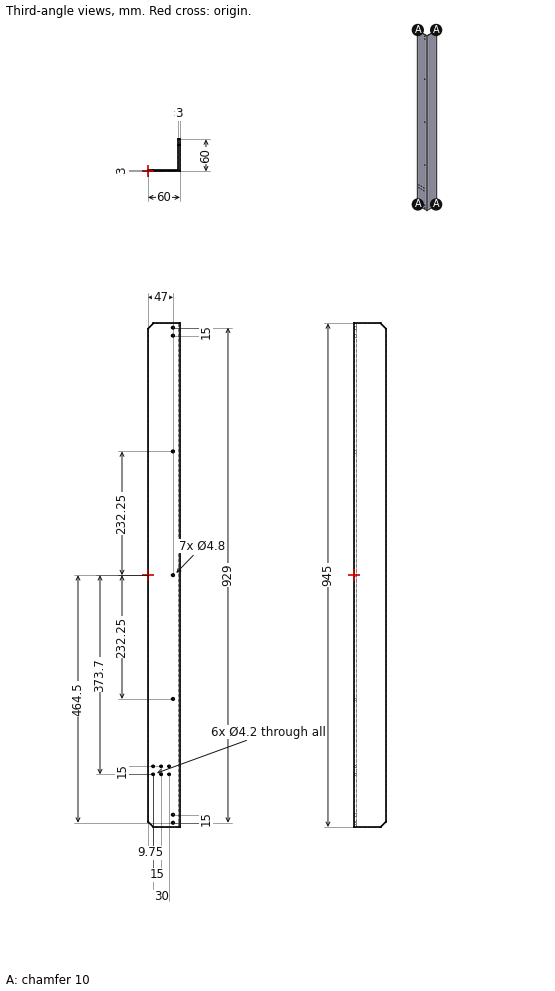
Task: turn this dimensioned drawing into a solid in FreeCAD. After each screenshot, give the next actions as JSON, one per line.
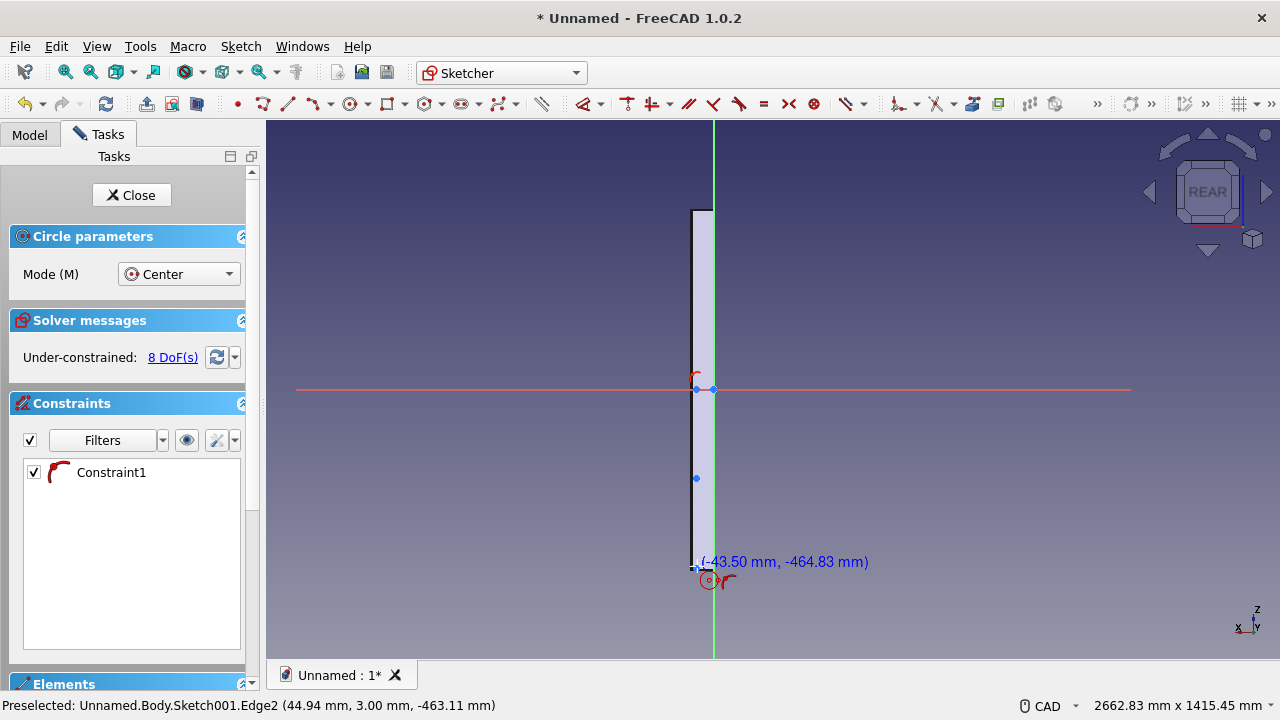
{"action": "scroll", "coordinate": [696, 213], "scroll_direction": "up", "scroll_amount": 17}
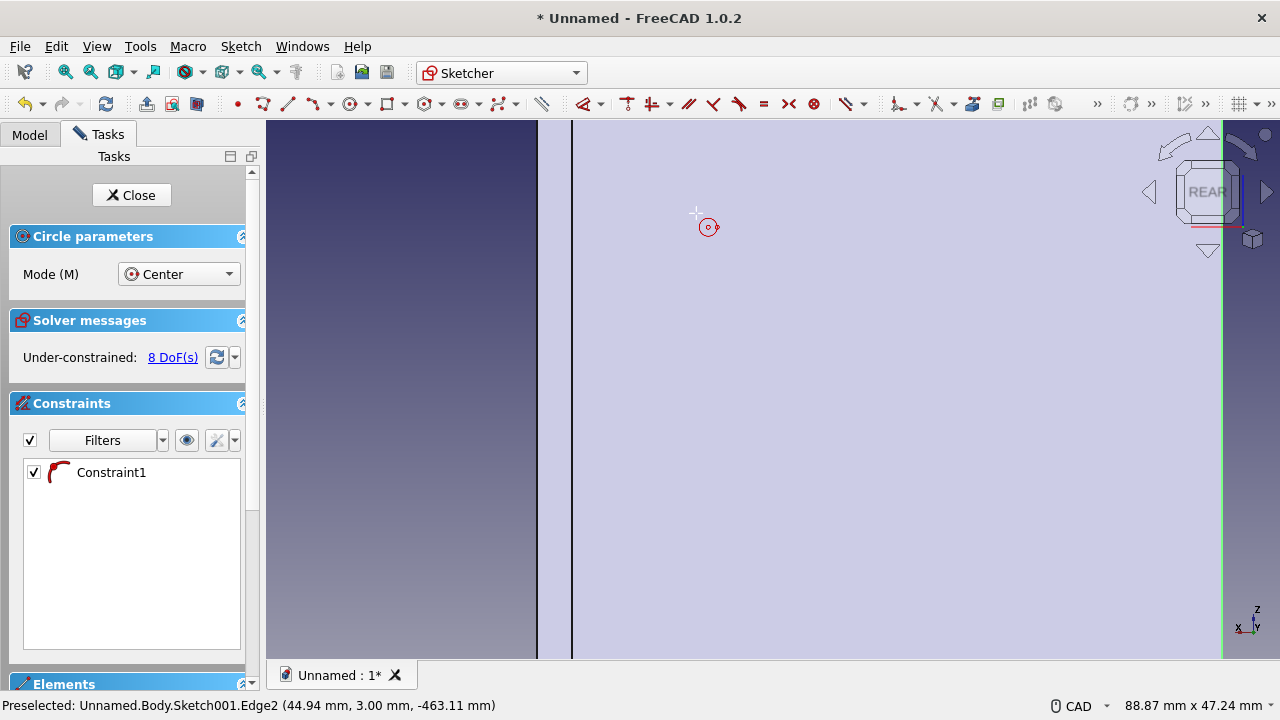
{"action": "scroll", "coordinate": [696, 213], "scroll_direction": "down", "scroll_amount": 17}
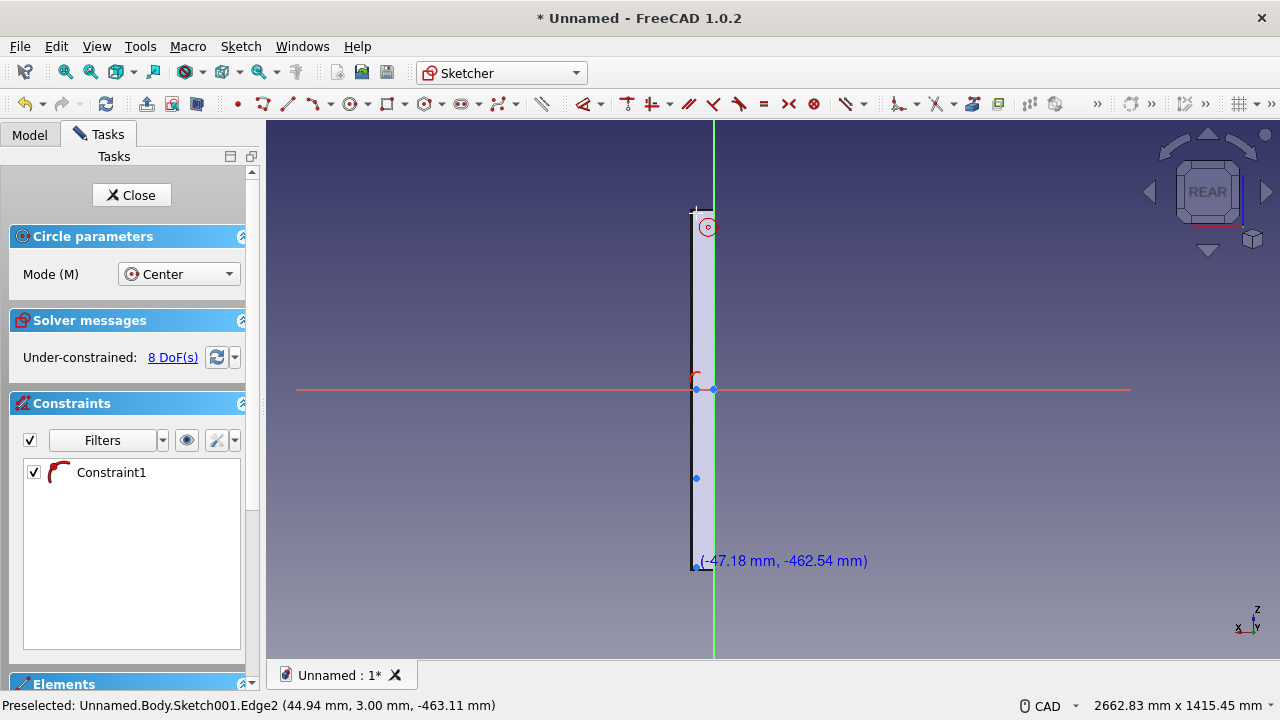
{"action": "left_click", "coordinate": [696, 213]}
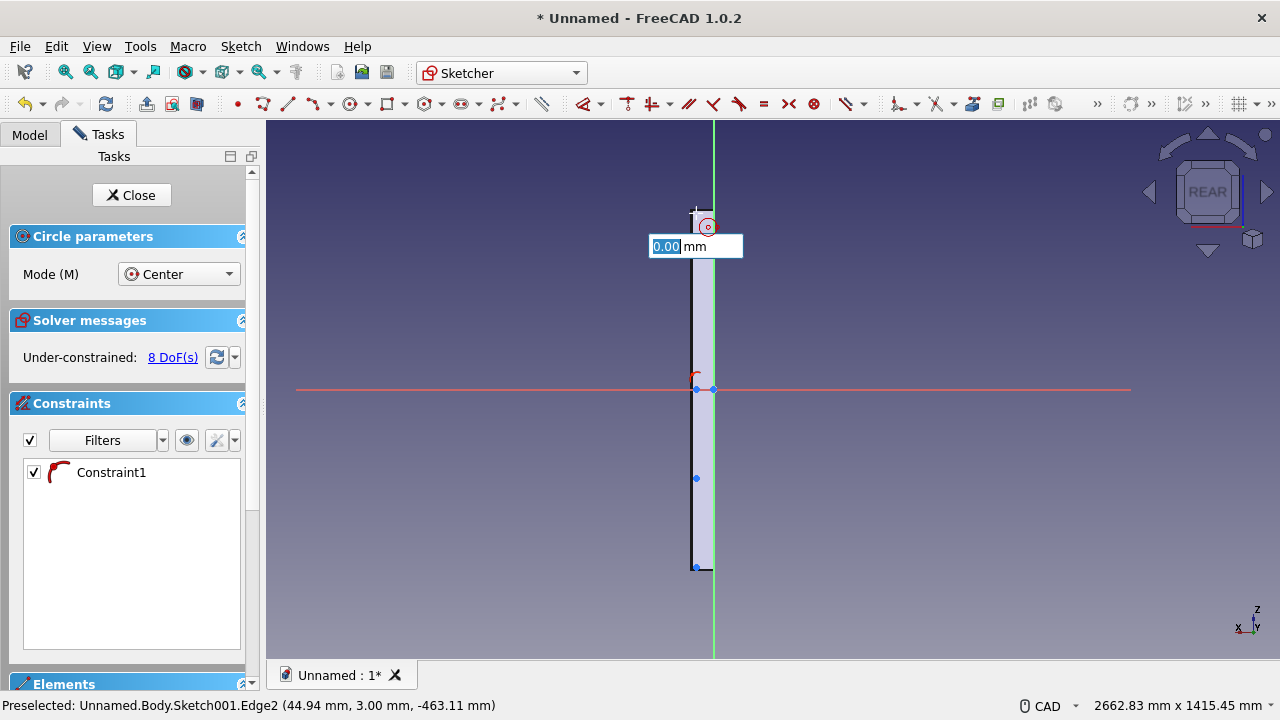
{"action": "scroll", "coordinate": [697, 212], "scroll_direction": "up", "scroll_amount": 15}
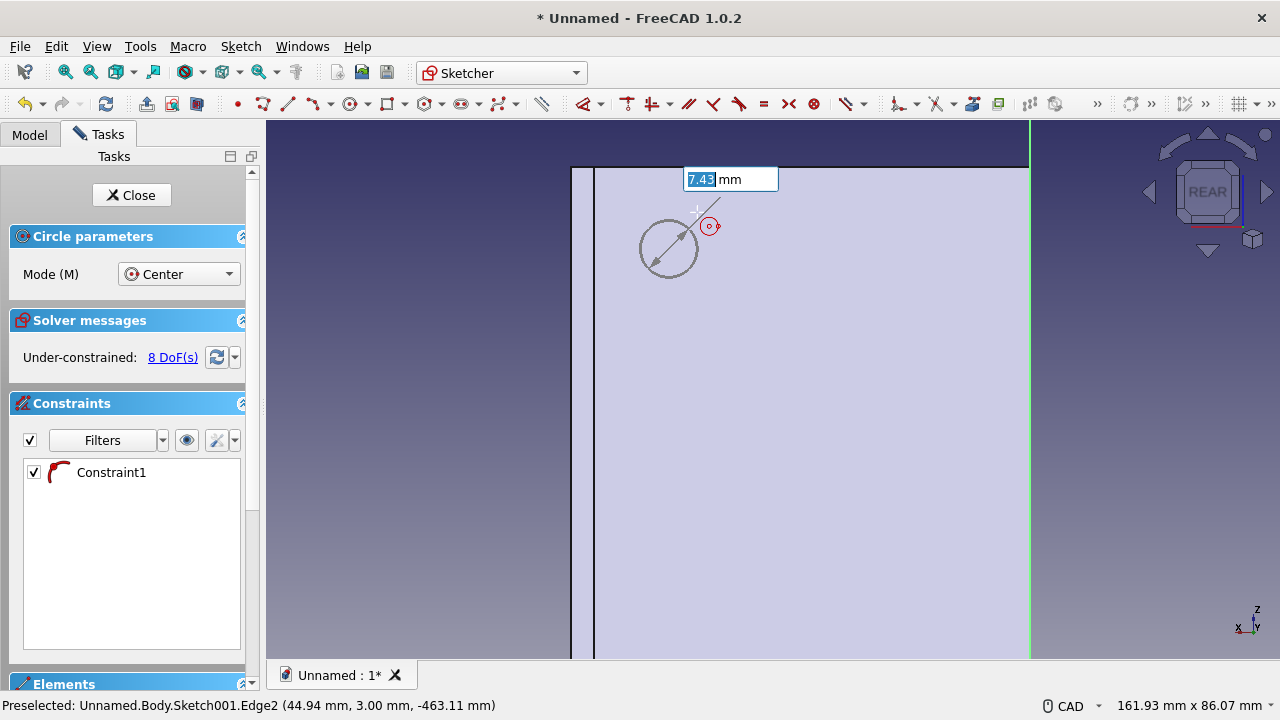
{"action": "left_click", "coordinate": [683, 215]}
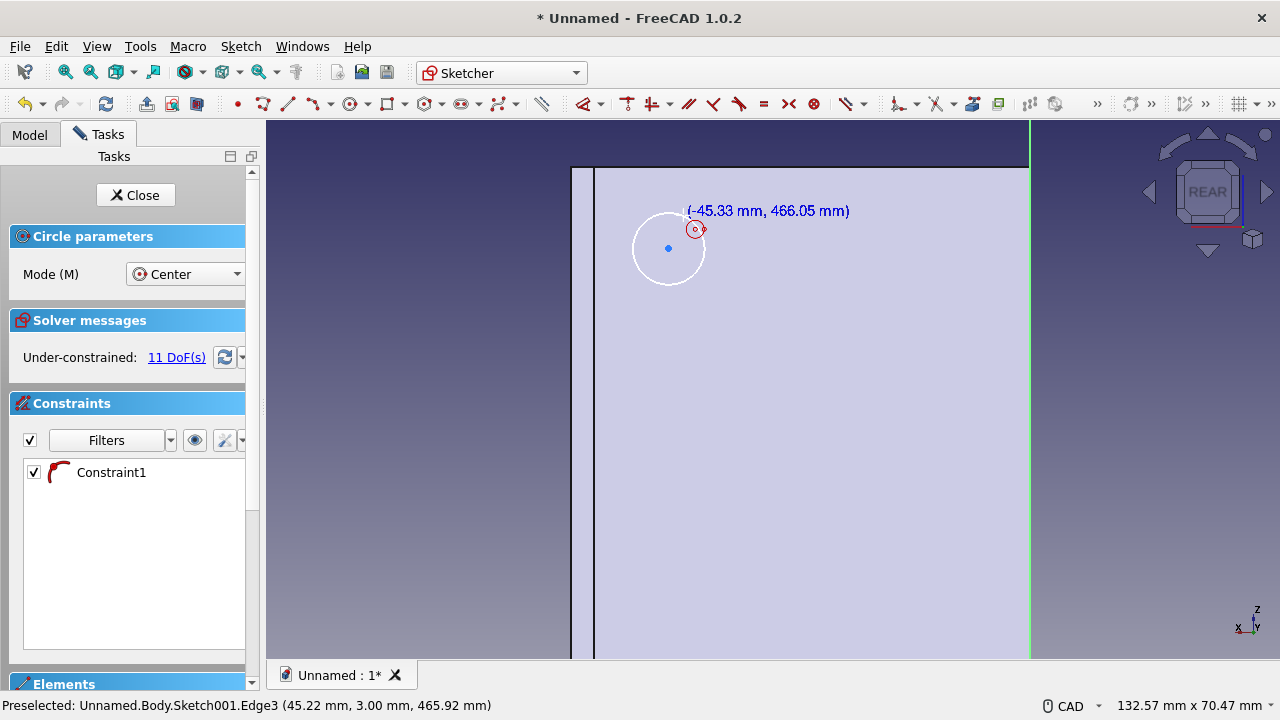
{"action": "scroll", "coordinate": [697, 212], "scroll_direction": "down", "scroll_amount": 15}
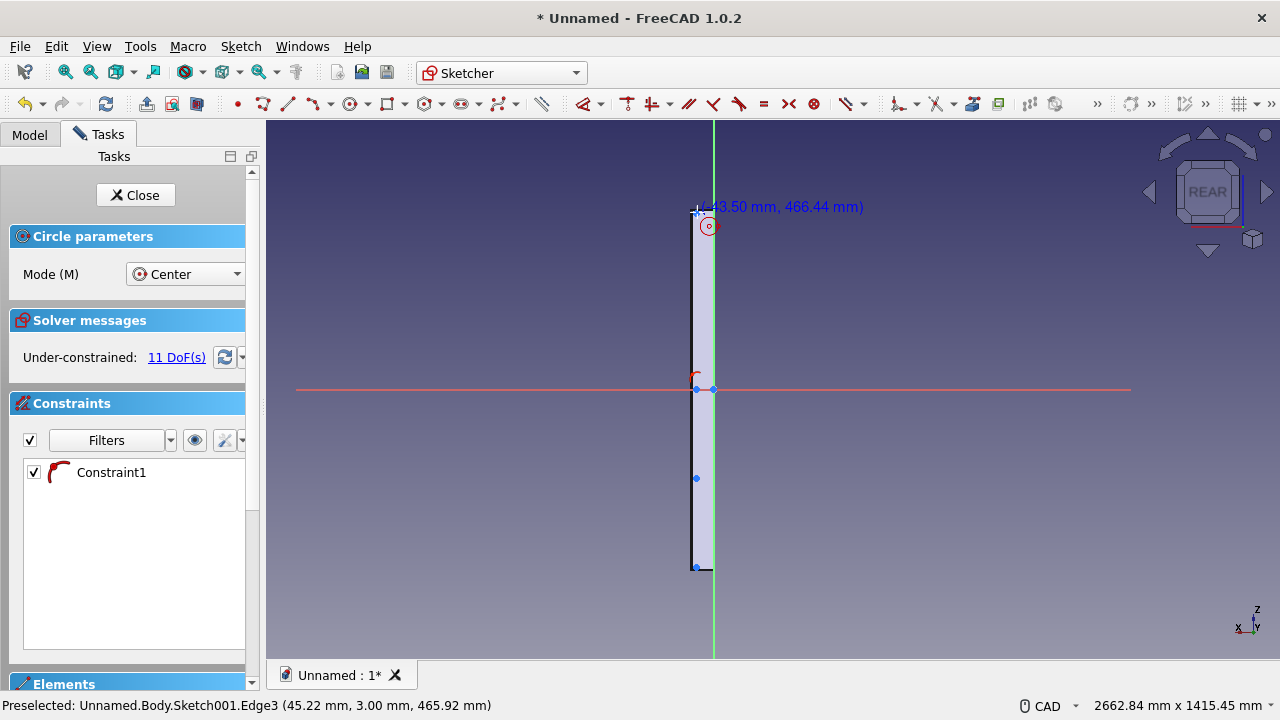
{"action": "scroll", "coordinate": [696, 301], "scroll_direction": "up", "scroll_amount": 17}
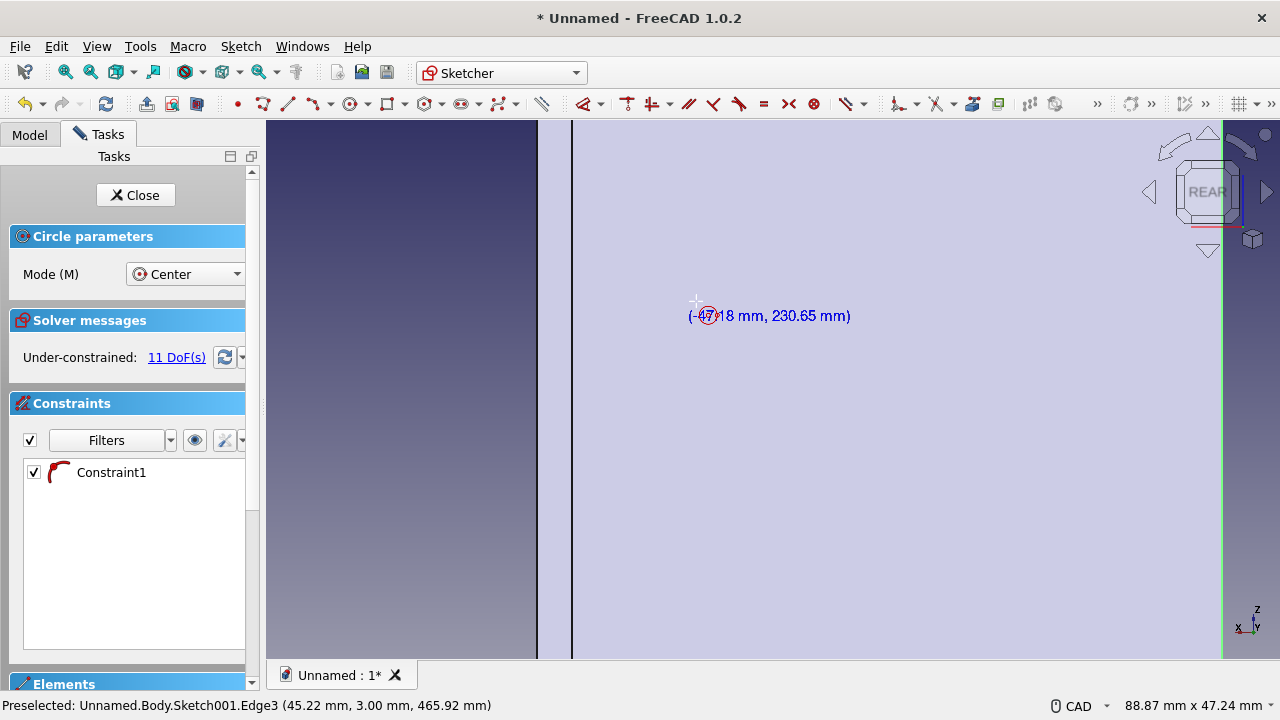
{"action": "scroll", "coordinate": [696, 301], "scroll_direction": "down", "scroll_amount": 17}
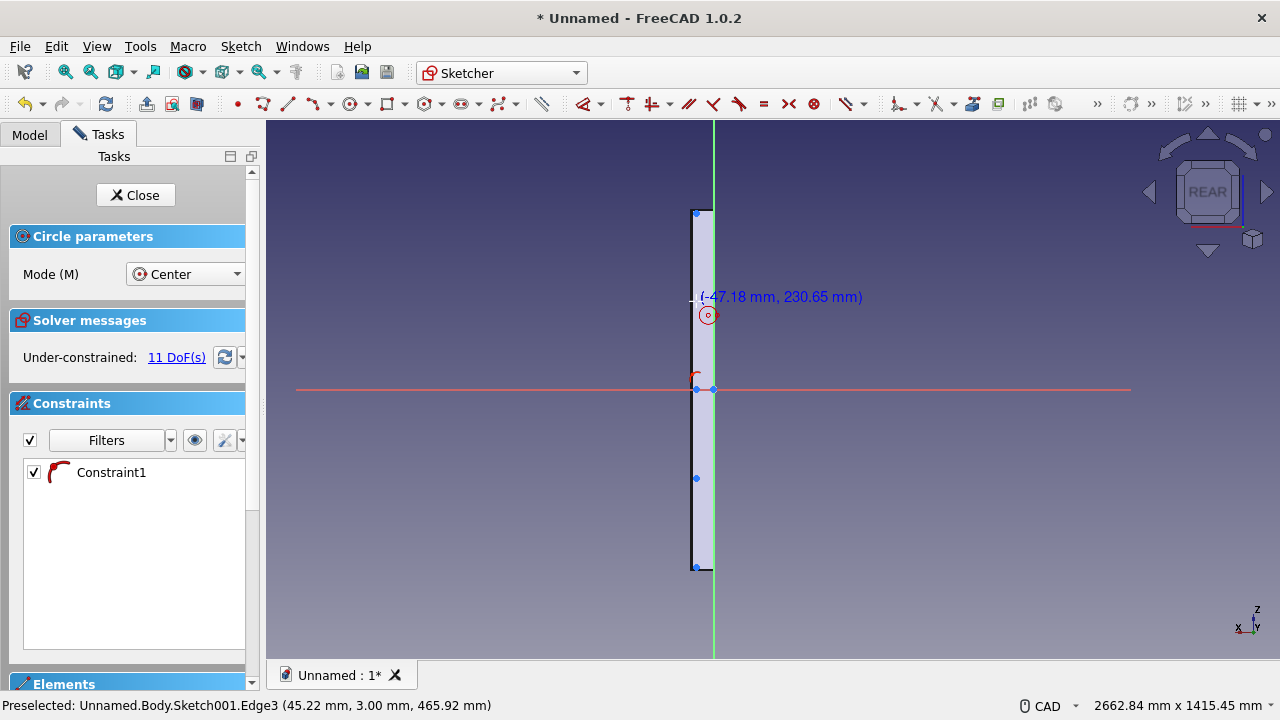
{"action": "left_click", "coordinate": [696, 301]}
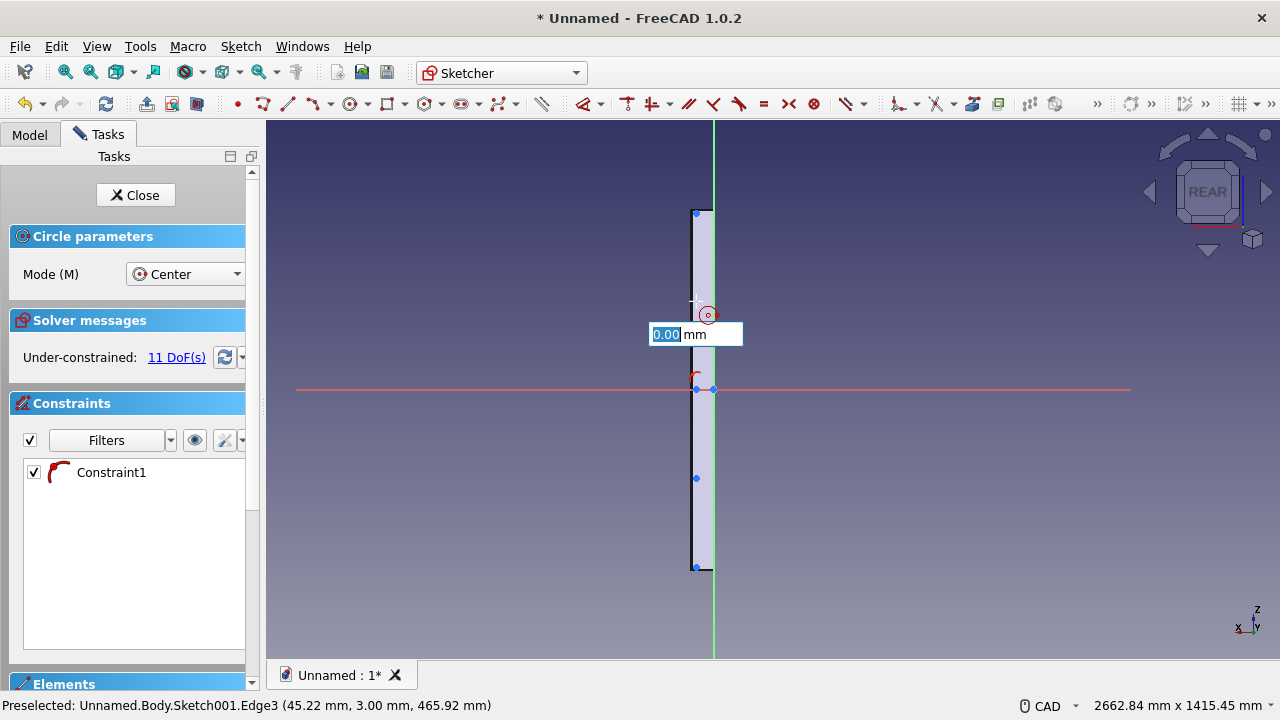
{"action": "scroll", "coordinate": [697, 301], "scroll_direction": "up", "scroll_amount": 15}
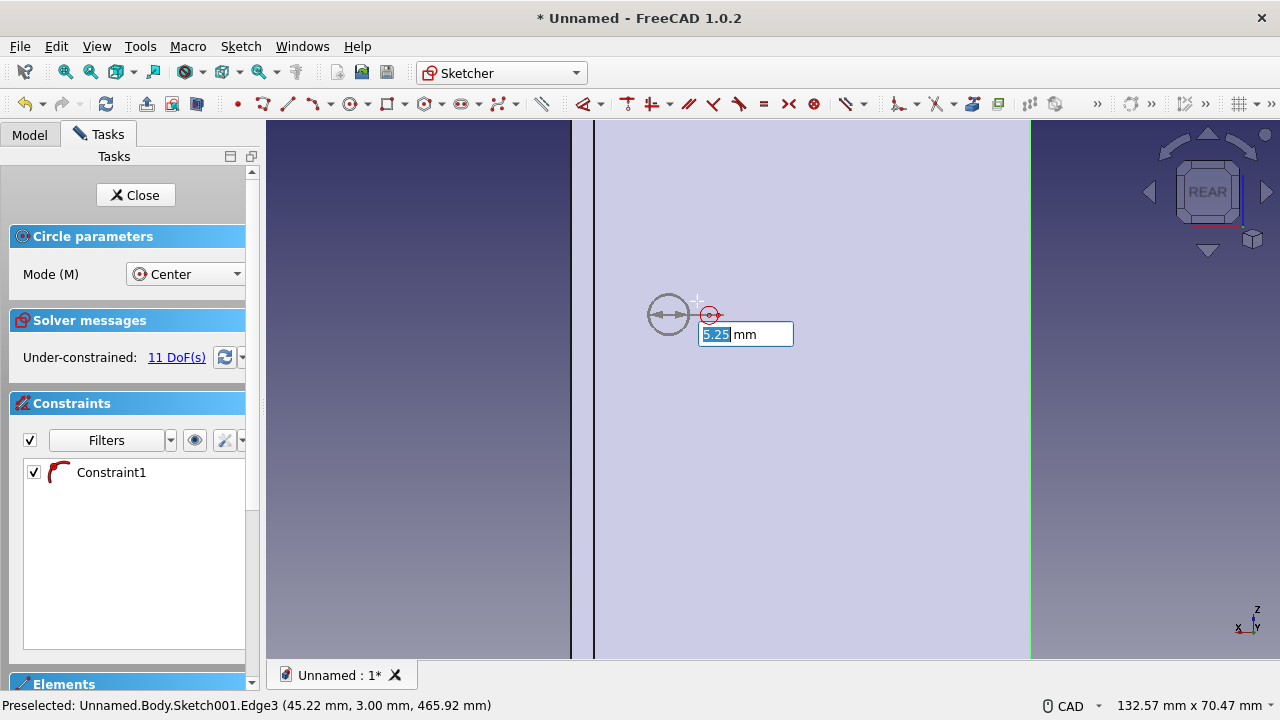
{"action": "left_click", "coordinate": [683, 289]}